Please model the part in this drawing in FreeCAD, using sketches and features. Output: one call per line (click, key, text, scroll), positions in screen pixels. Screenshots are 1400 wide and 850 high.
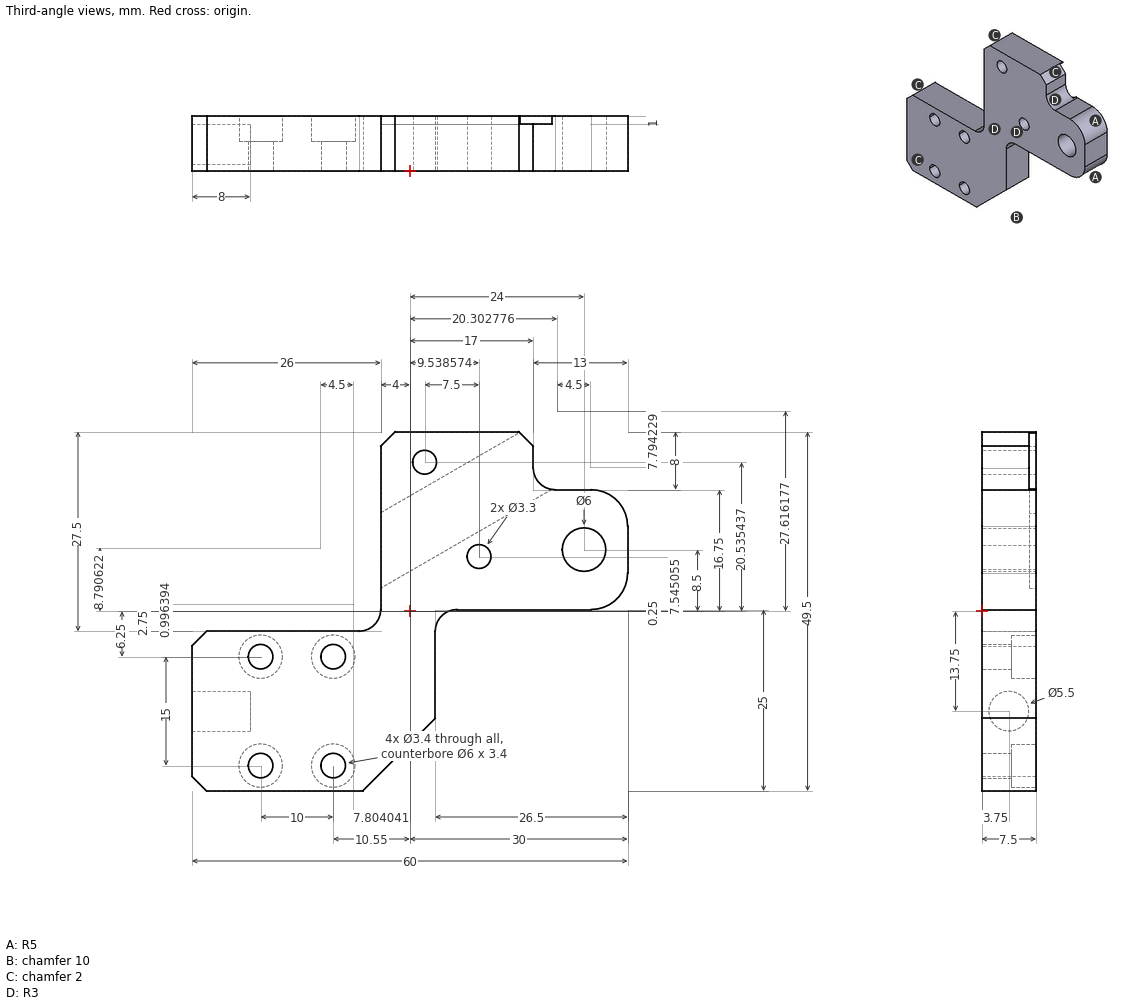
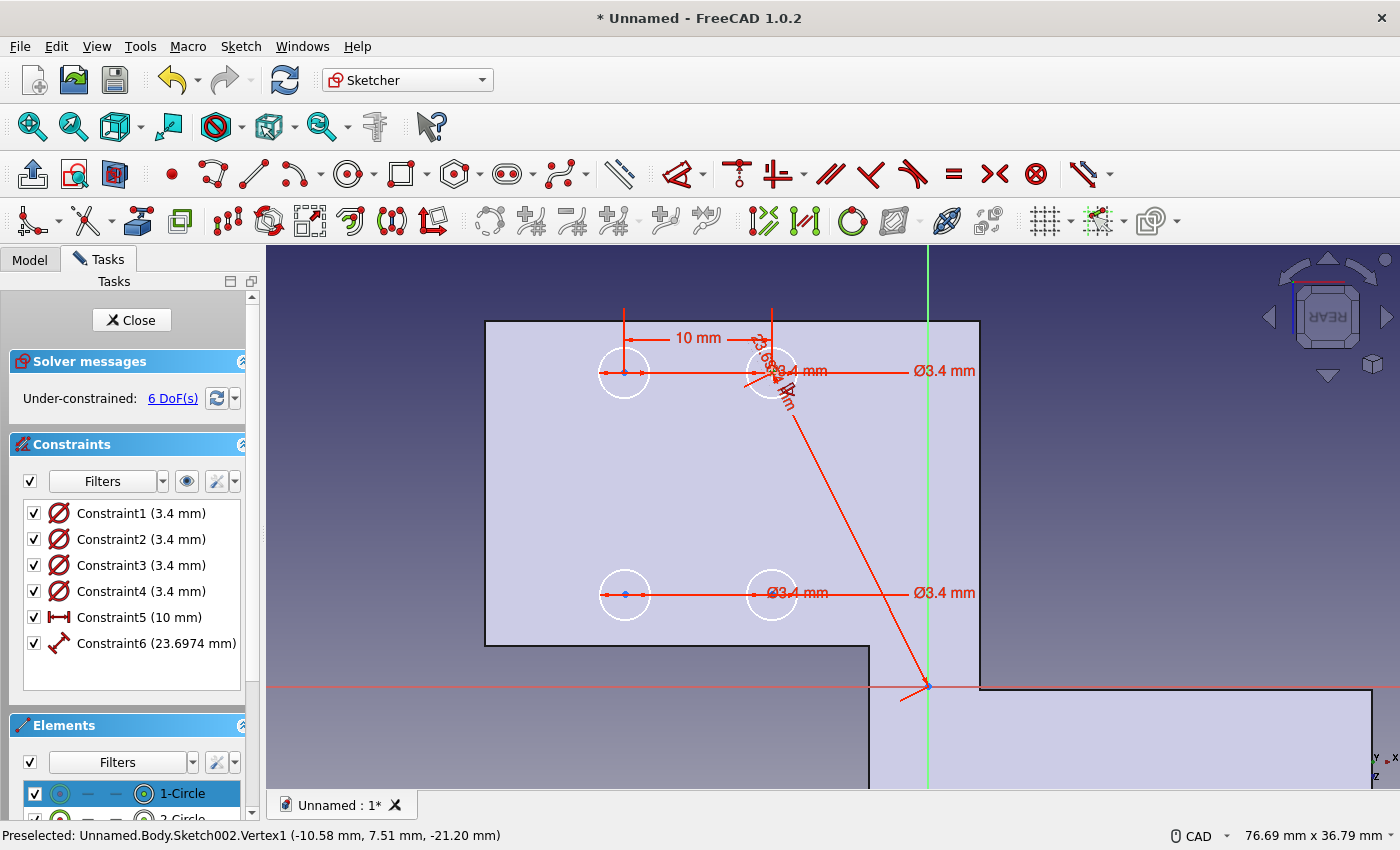
click(625, 595)
click(699, 629)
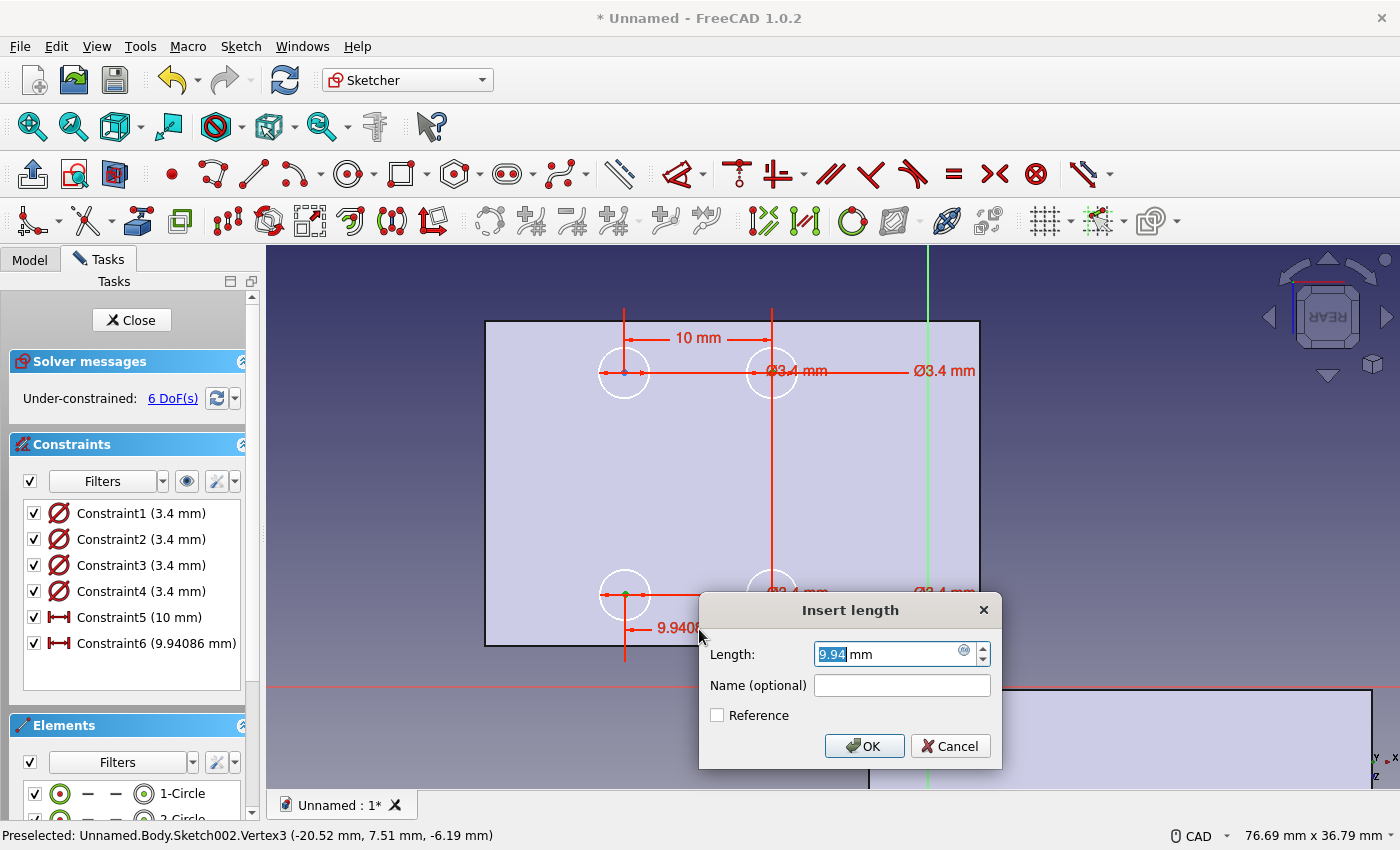
text(10)
key(Return)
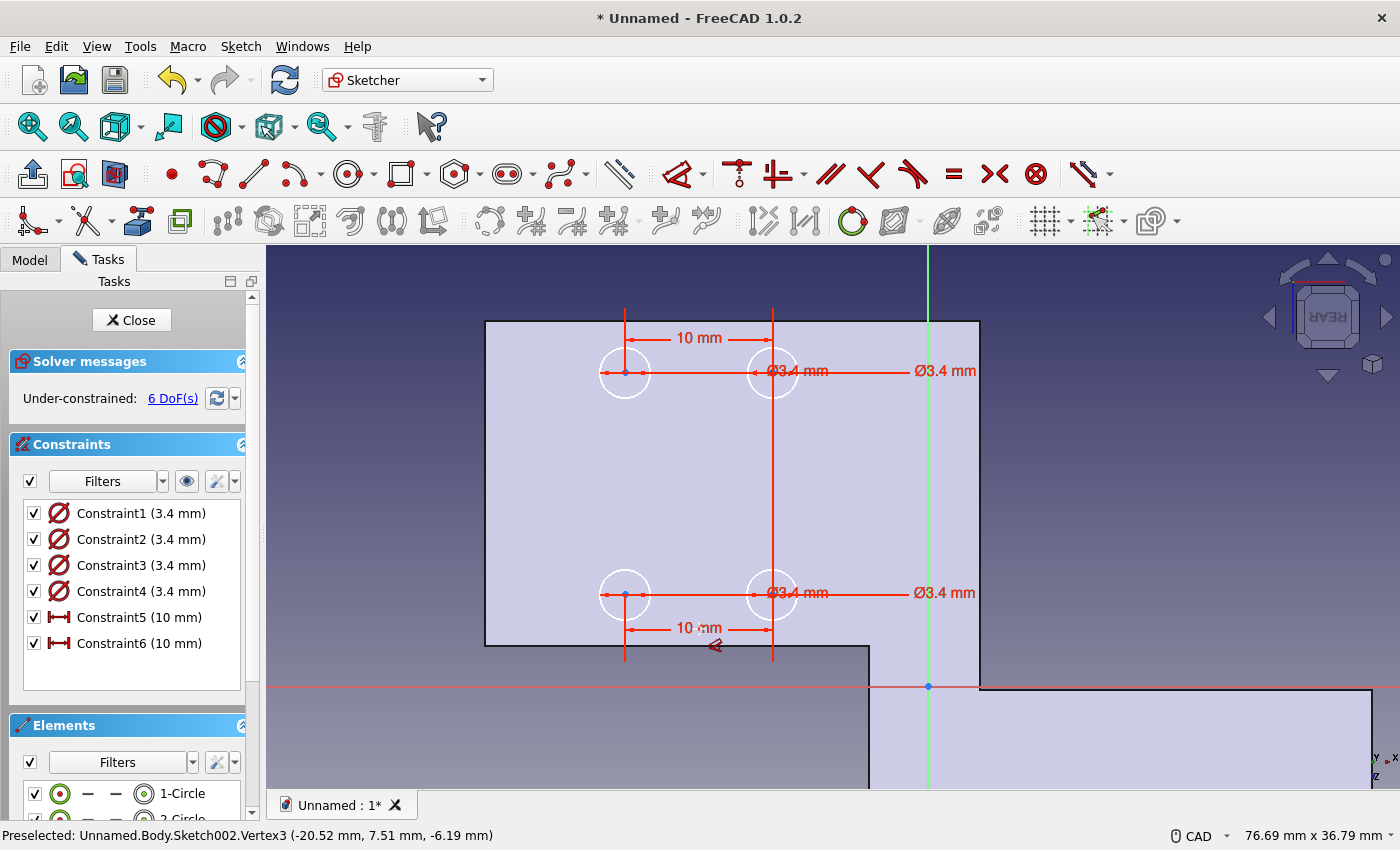
click(625, 373)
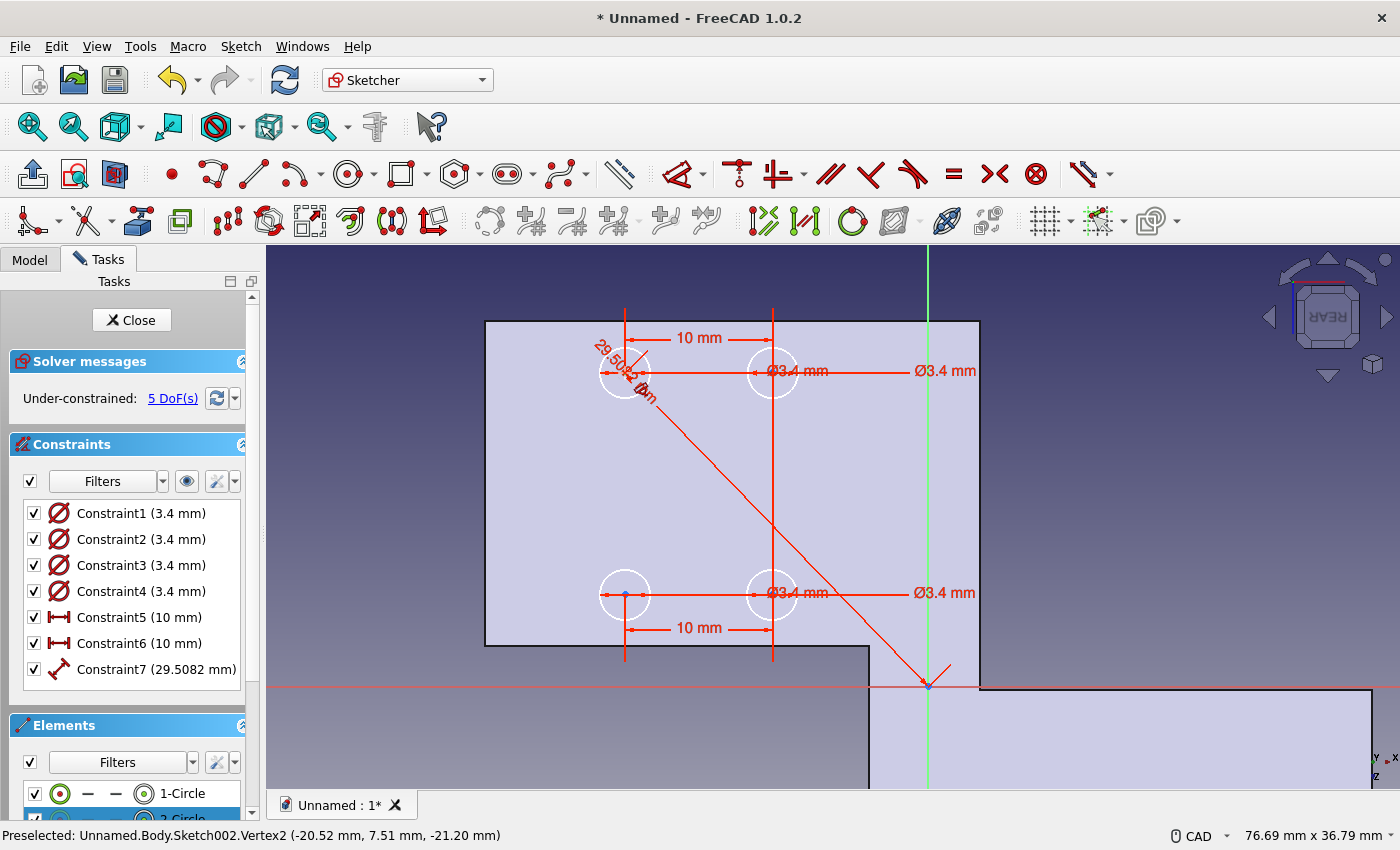
click(625, 595)
click(591, 484)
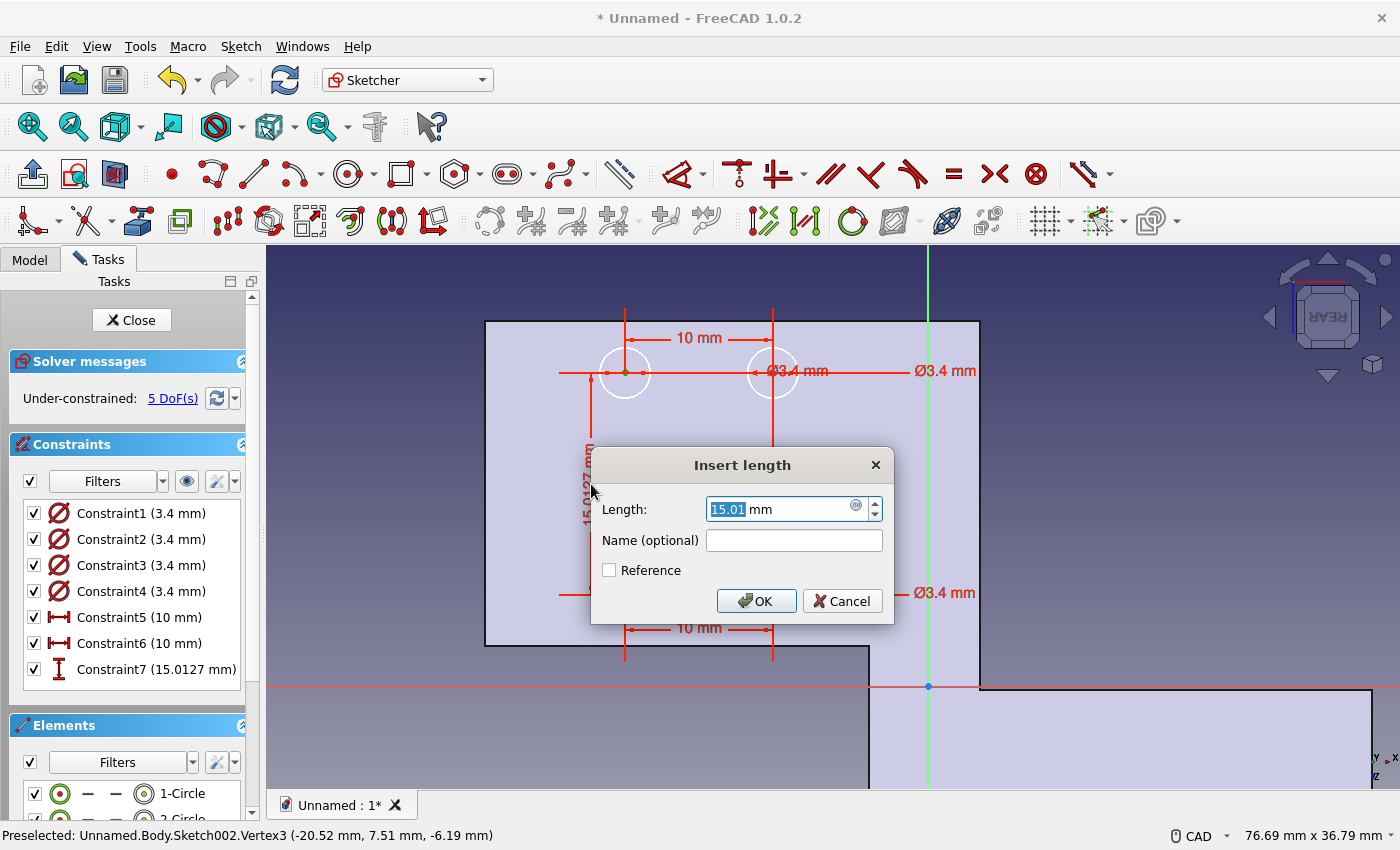
text(15)
key(Return)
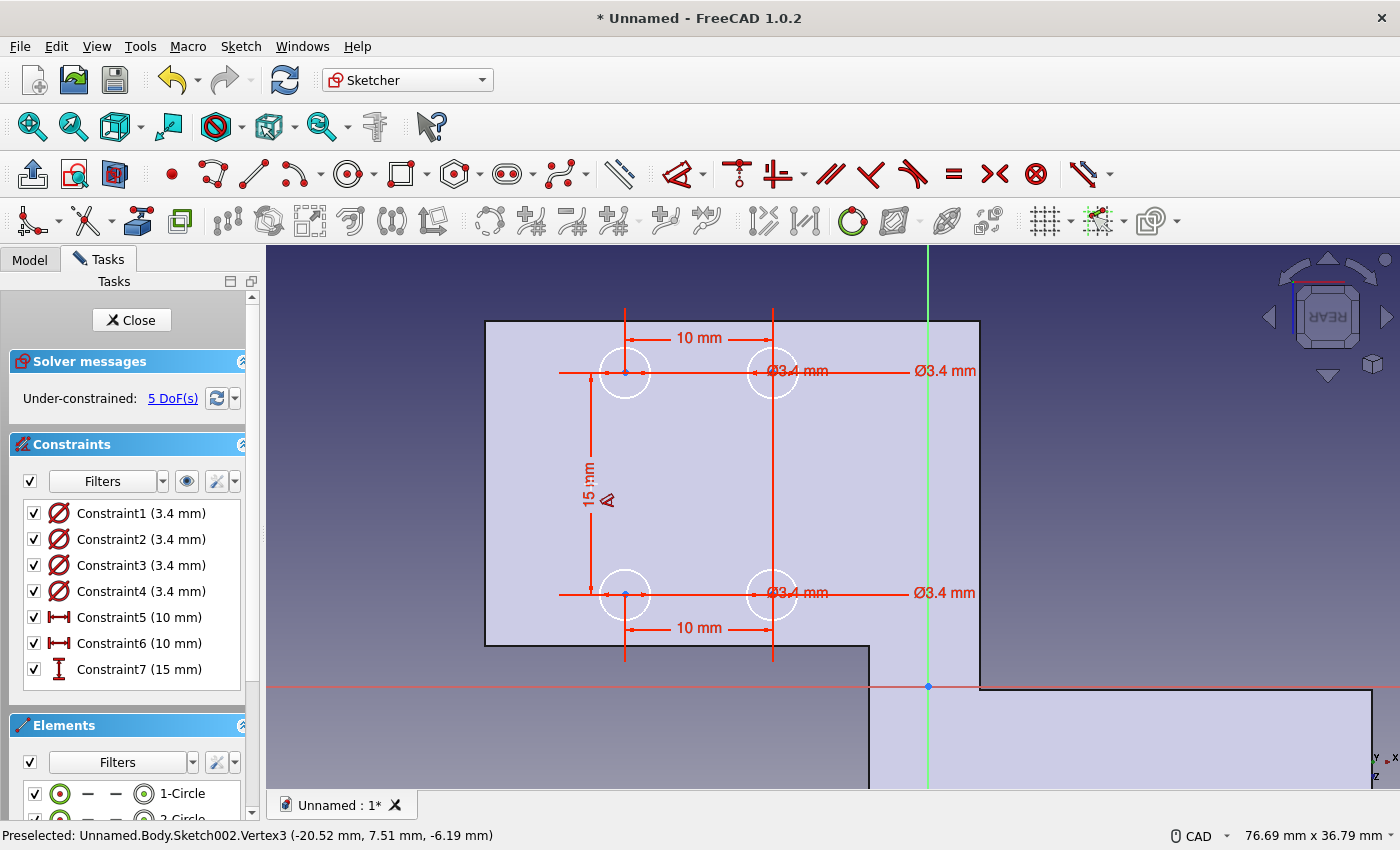
click(773, 373)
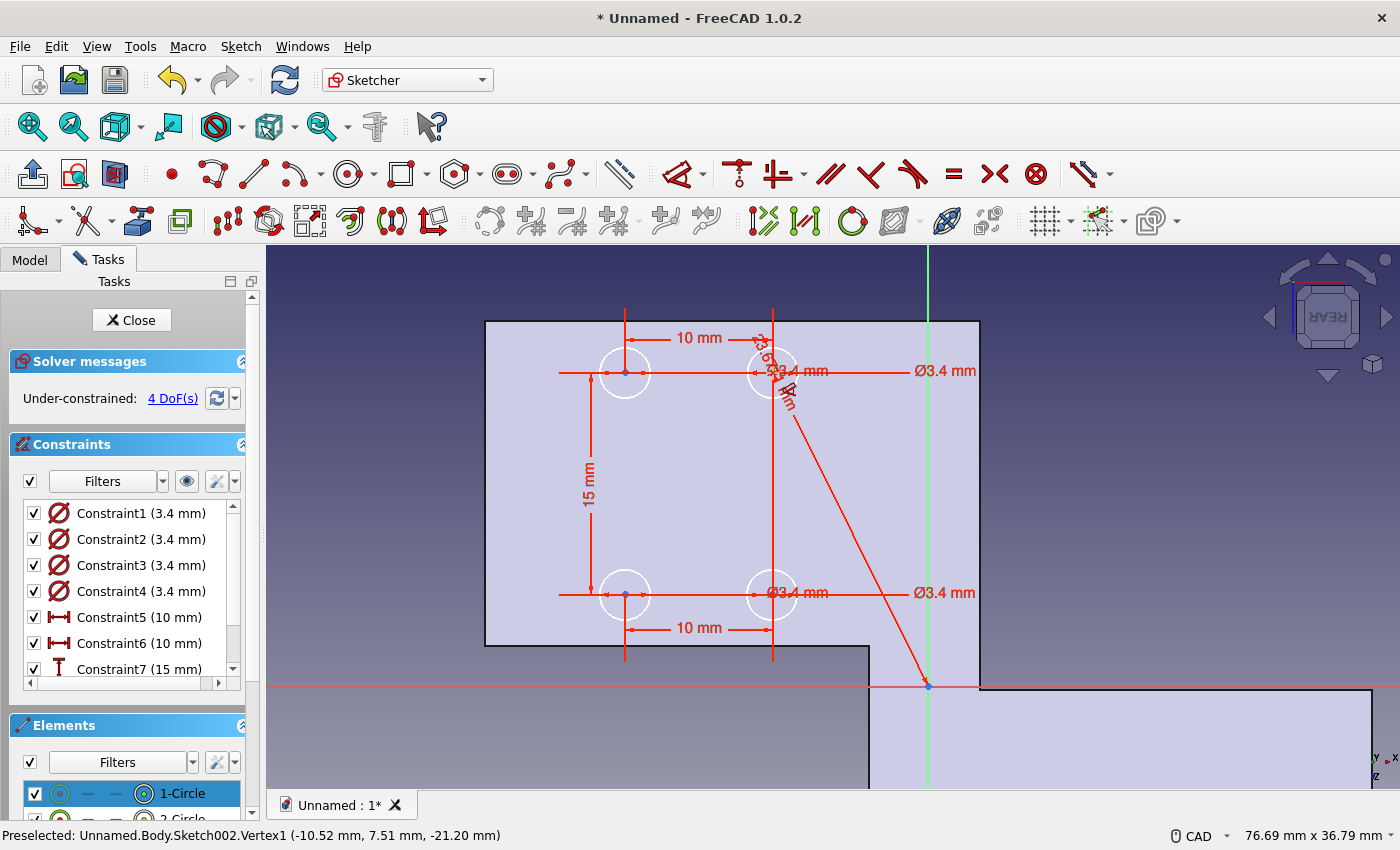
click(625, 595)
click(591, 433)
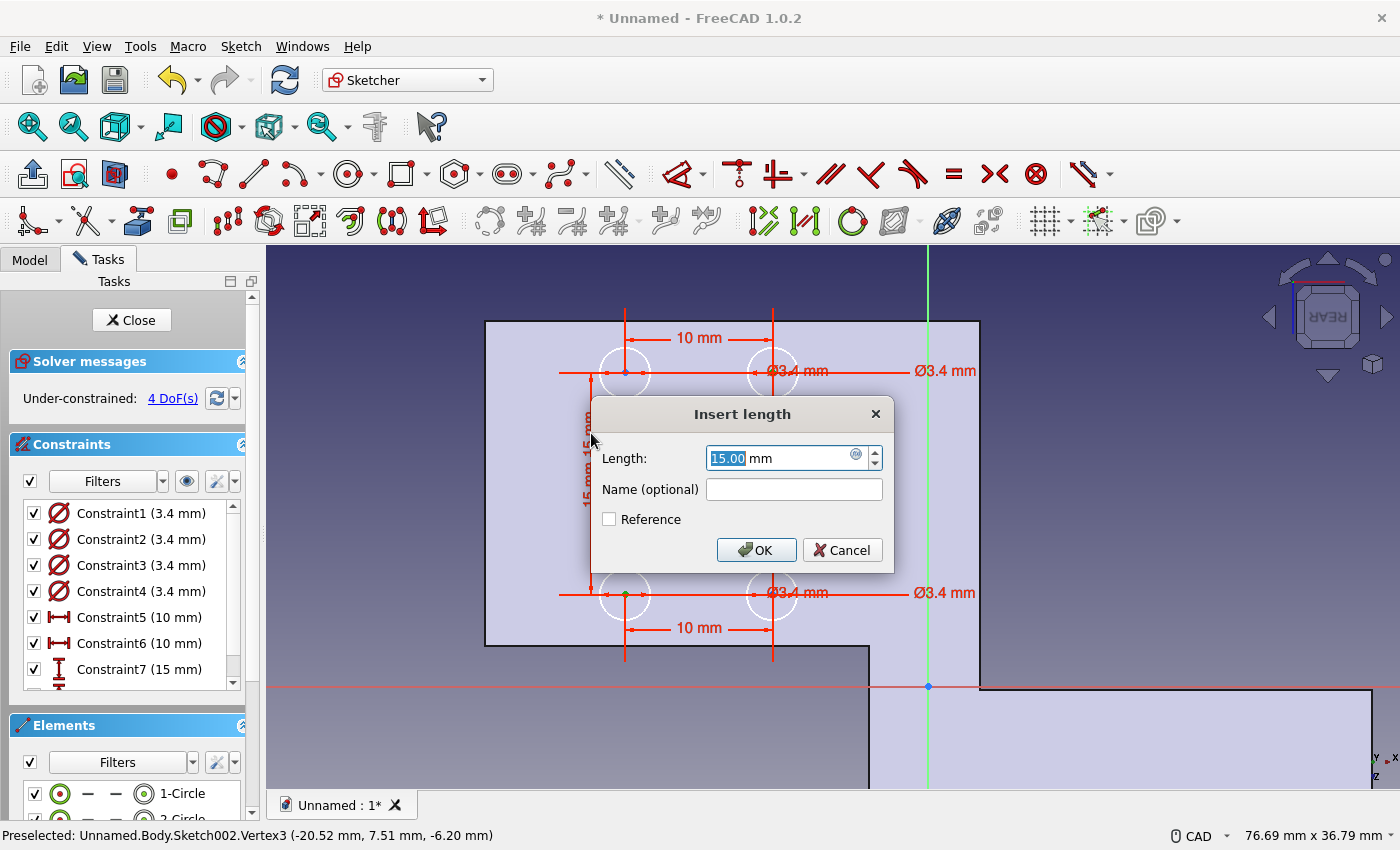
text(15)
key(Return)